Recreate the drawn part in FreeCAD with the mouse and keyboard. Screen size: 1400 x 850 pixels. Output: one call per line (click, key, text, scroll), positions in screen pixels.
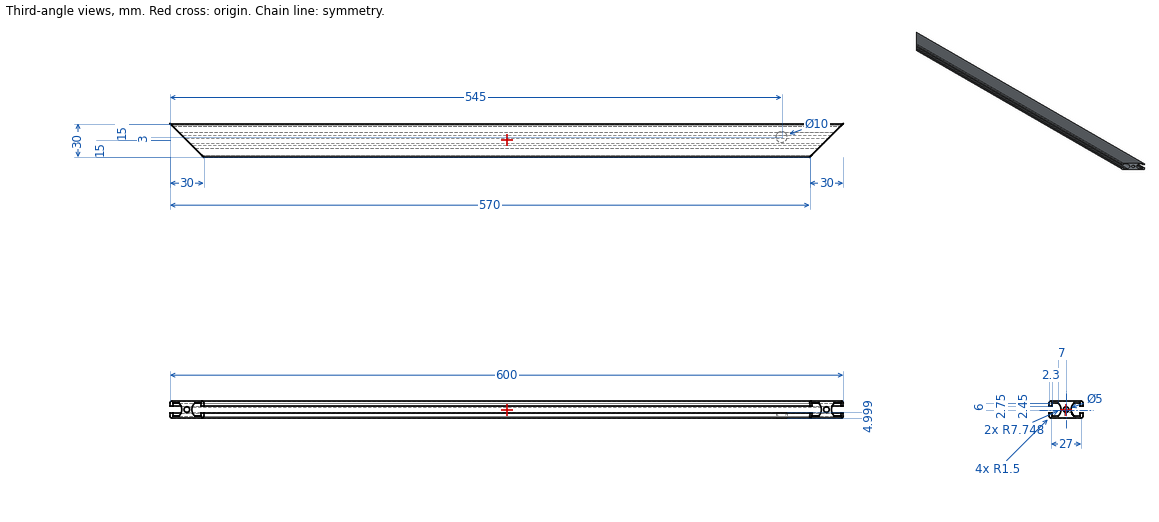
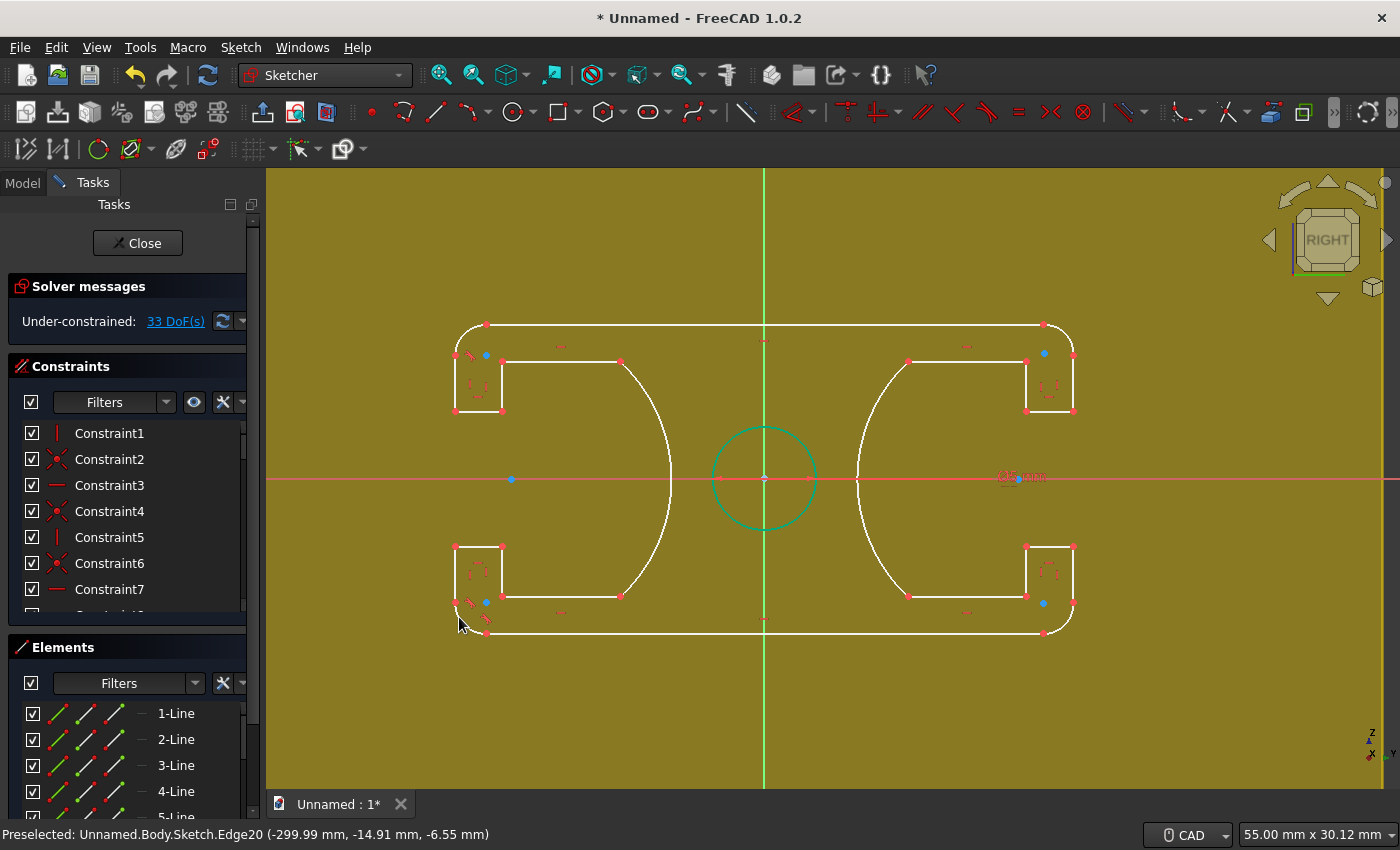
click(653, 634)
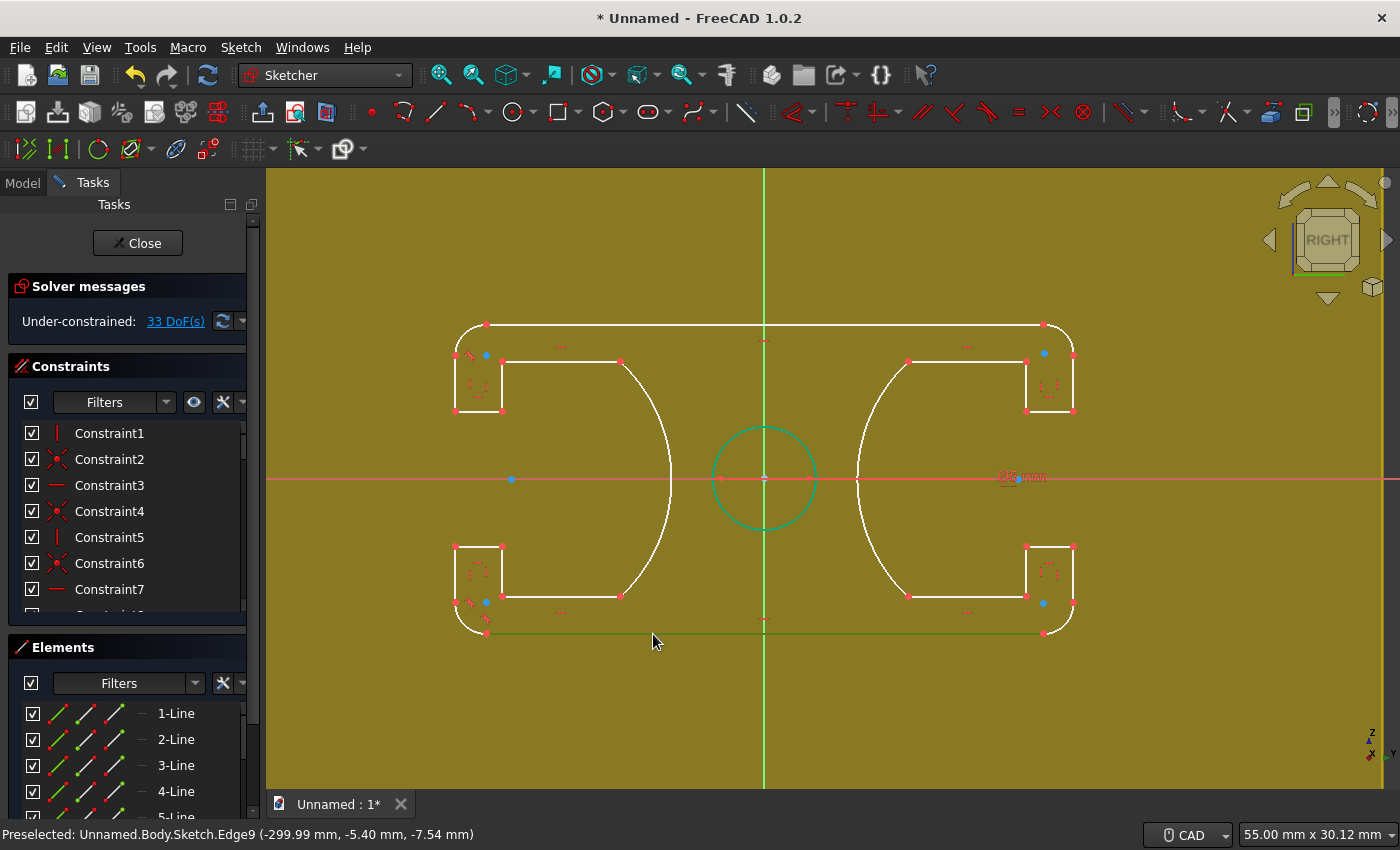
click(1057, 631)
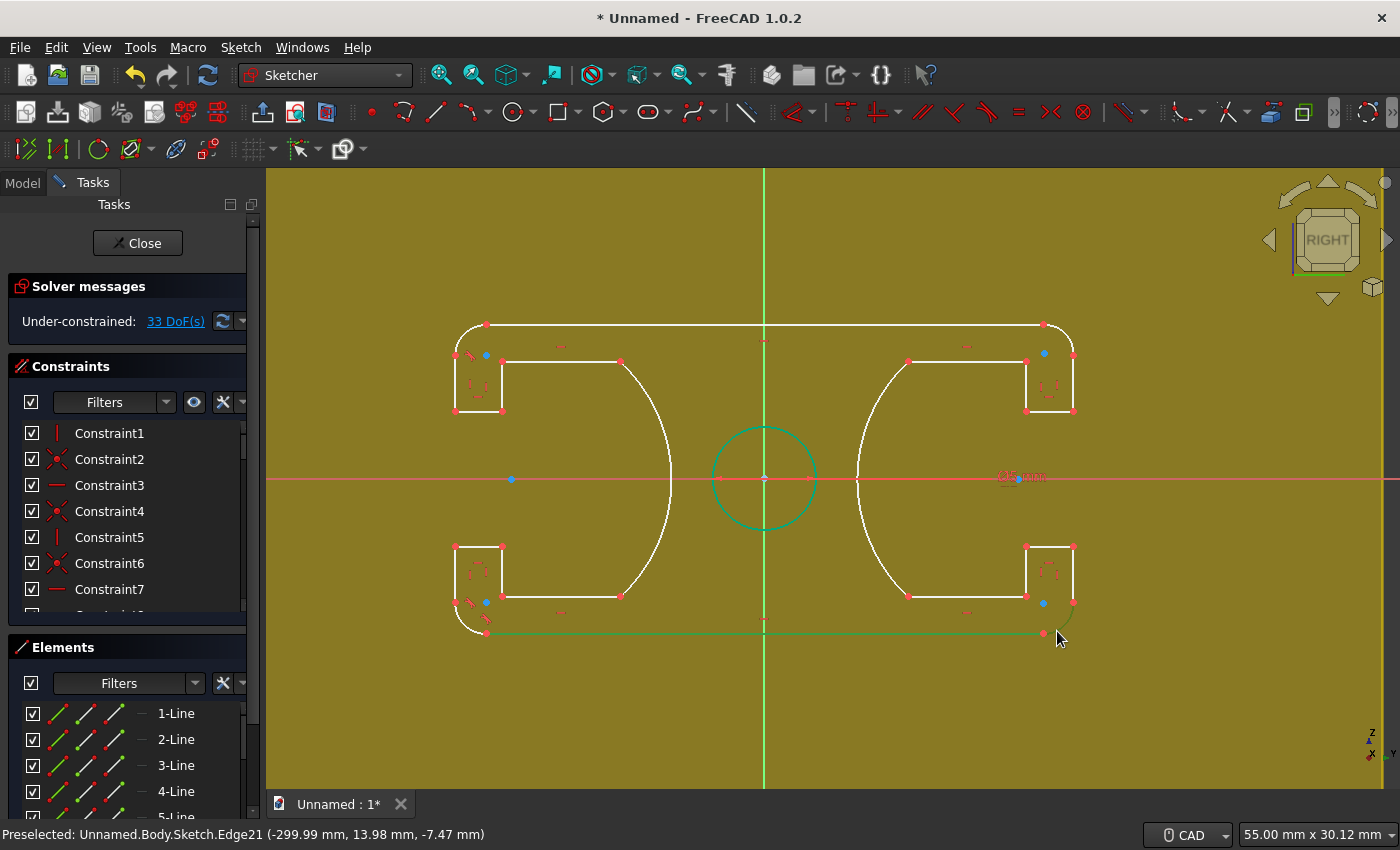
key(t)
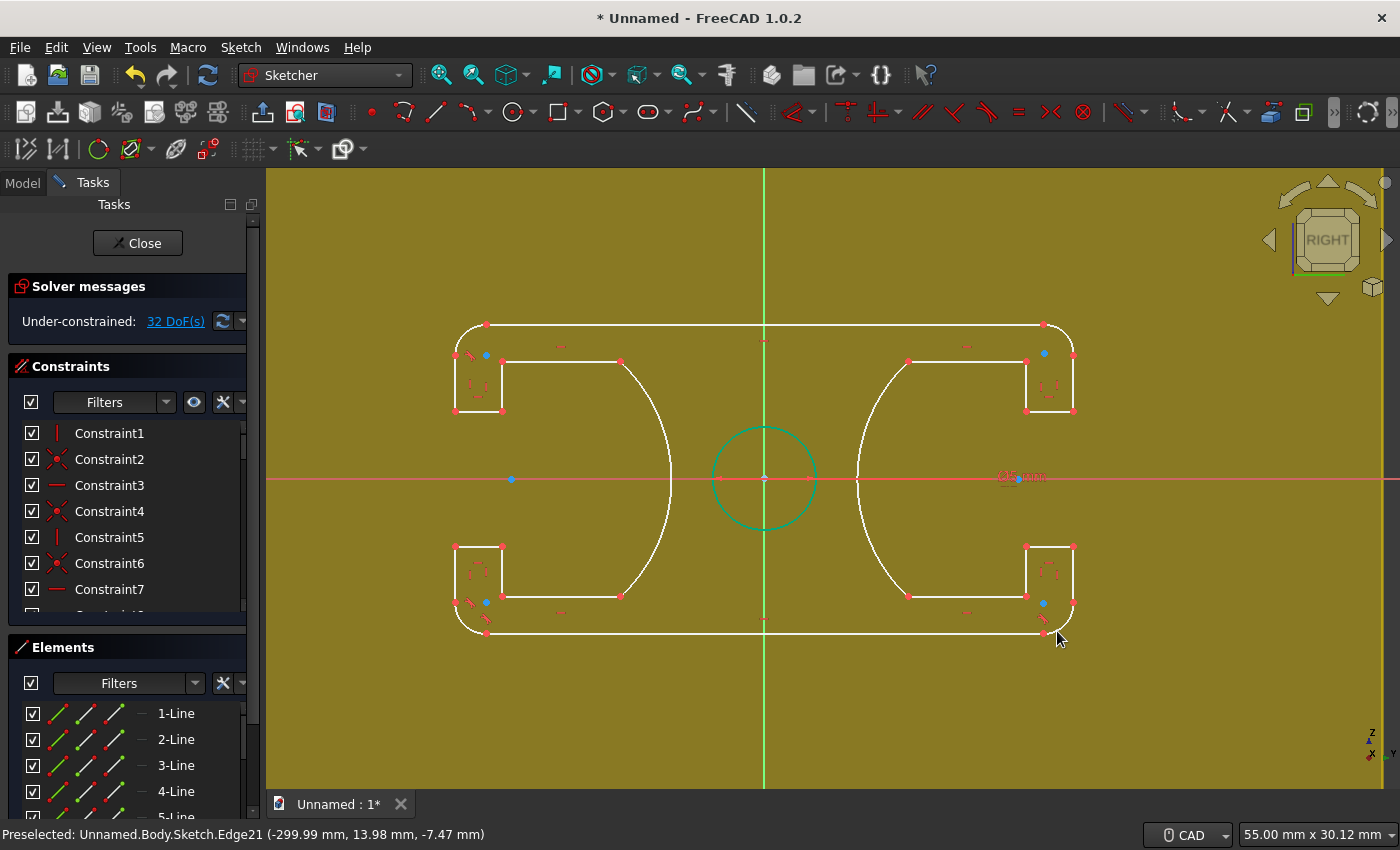
click(1073, 586)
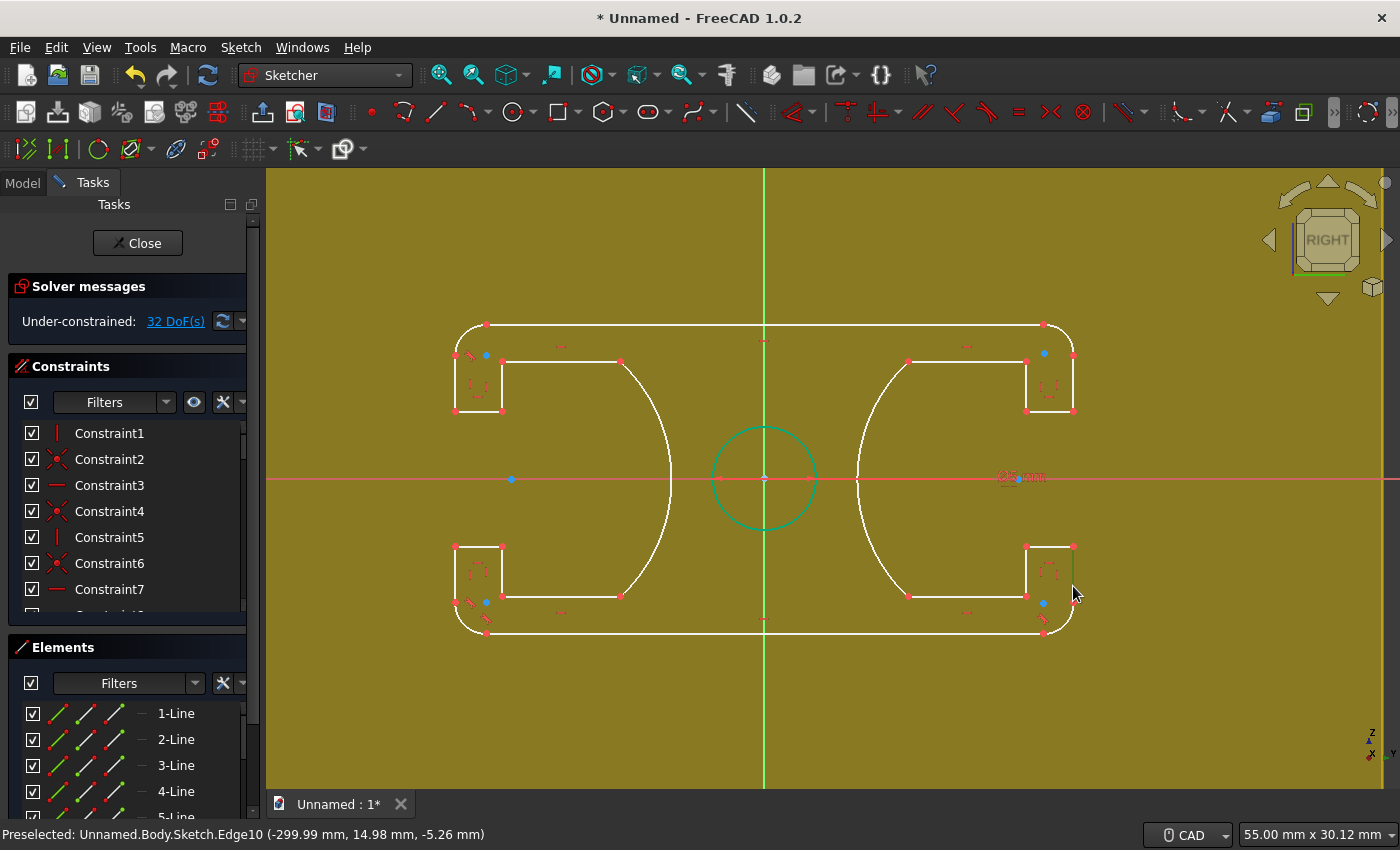
click(1057, 631)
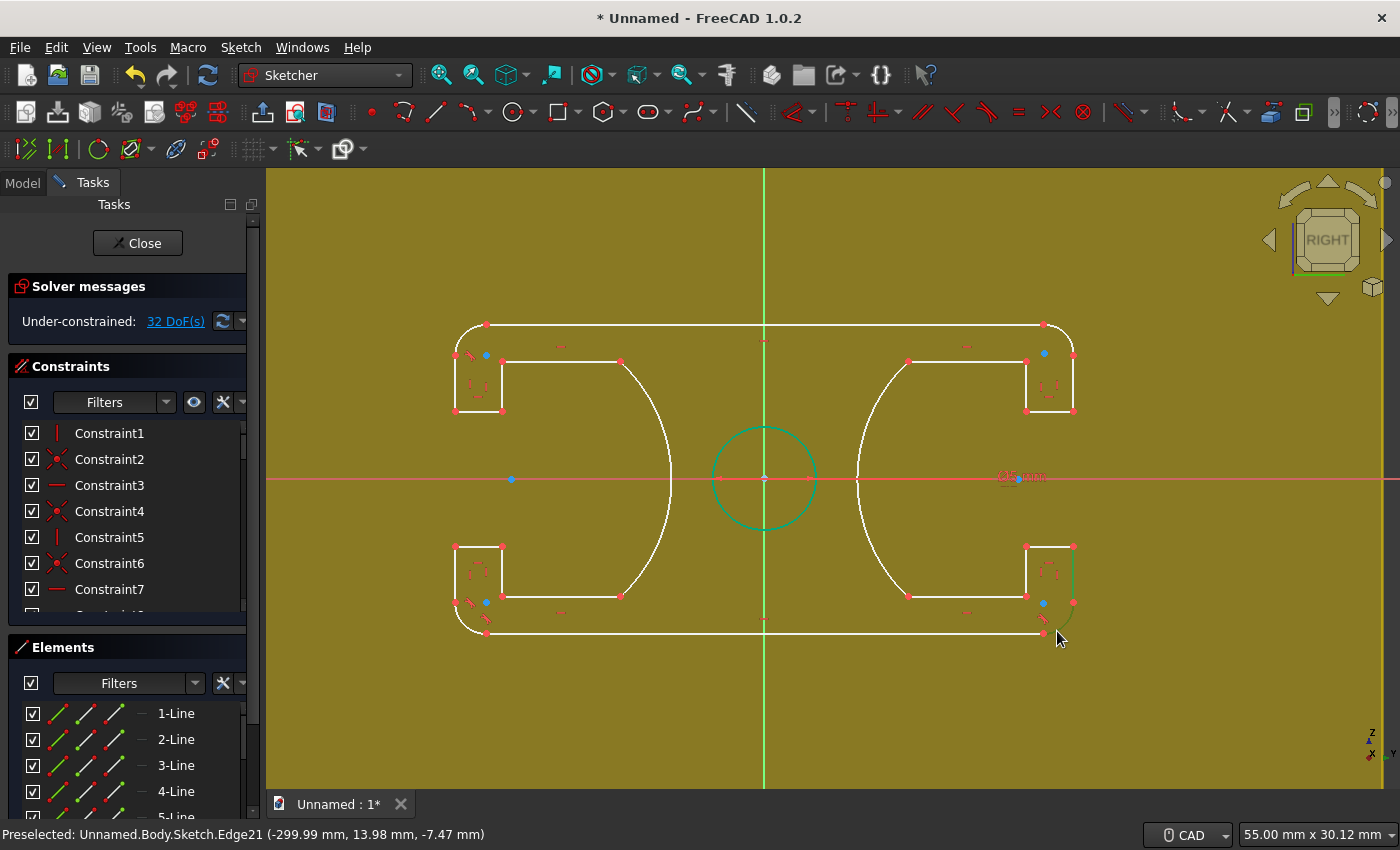
key(t)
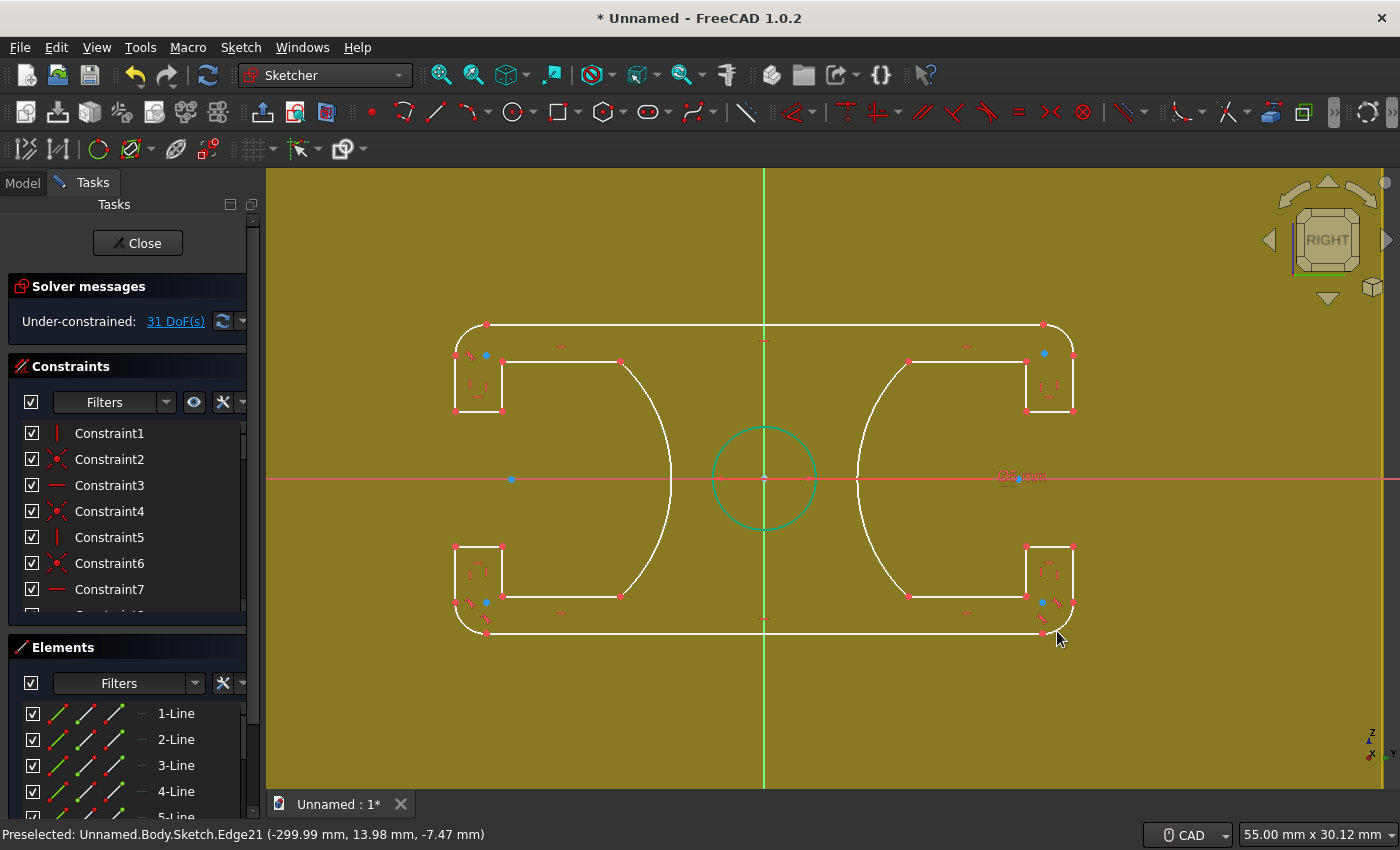
click(1073, 395)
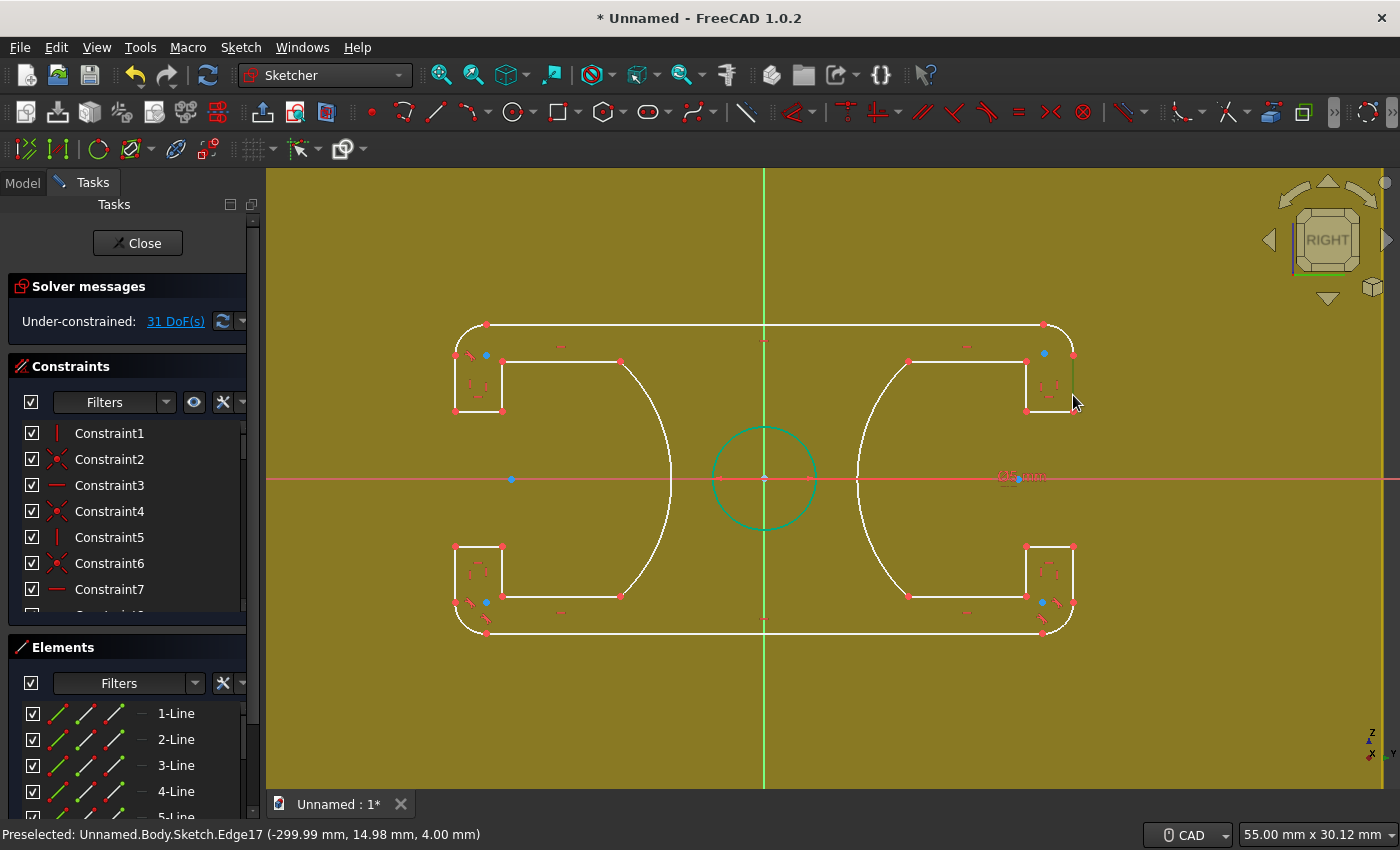
click(1071, 342)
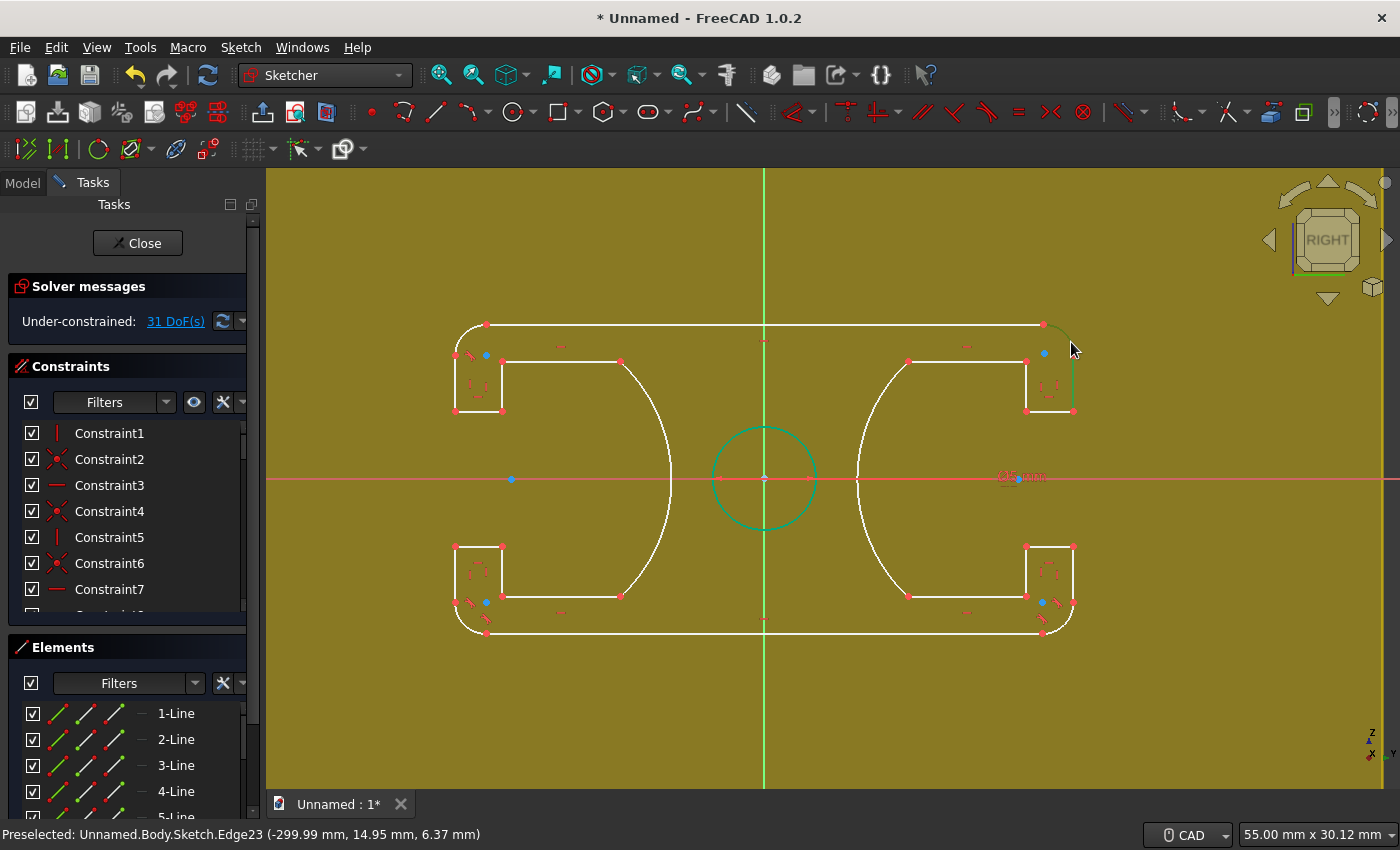
key(t)